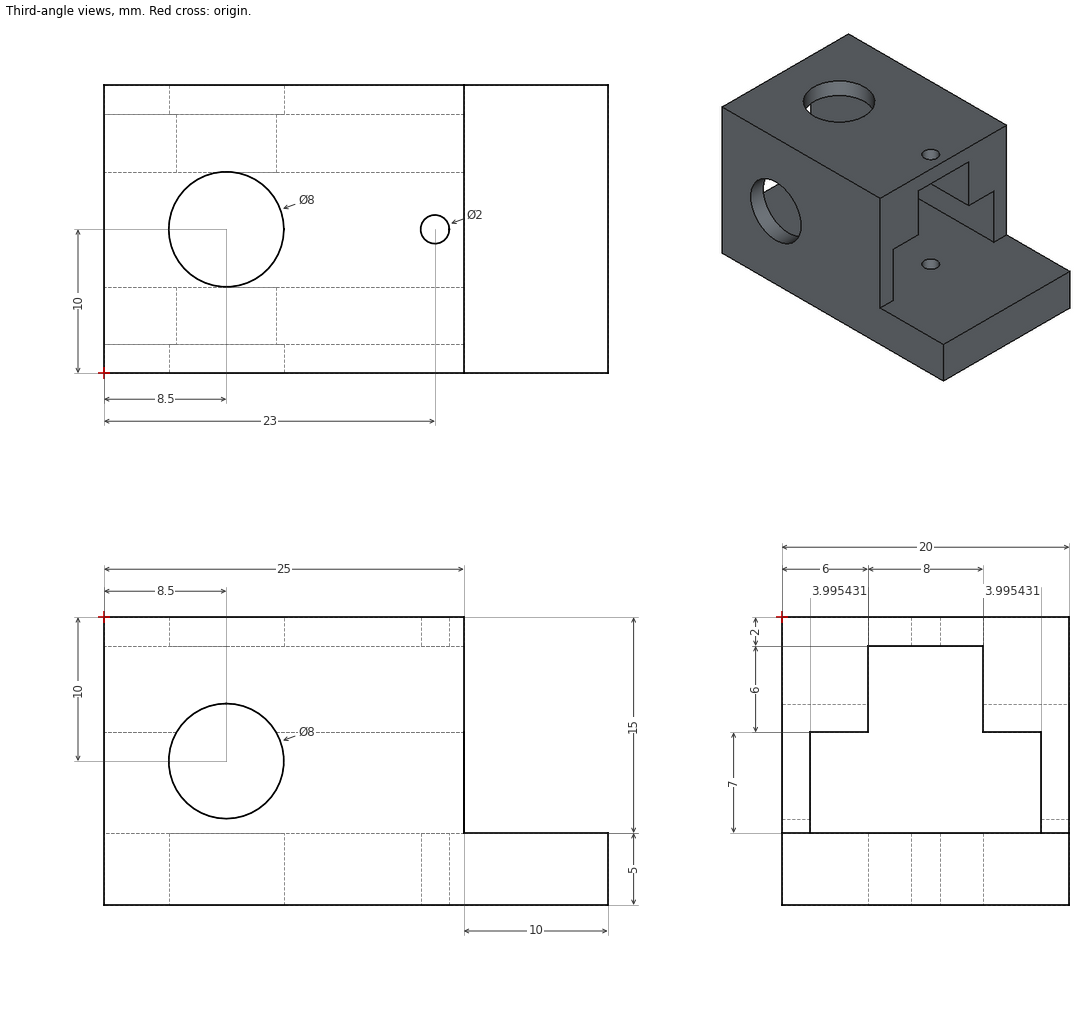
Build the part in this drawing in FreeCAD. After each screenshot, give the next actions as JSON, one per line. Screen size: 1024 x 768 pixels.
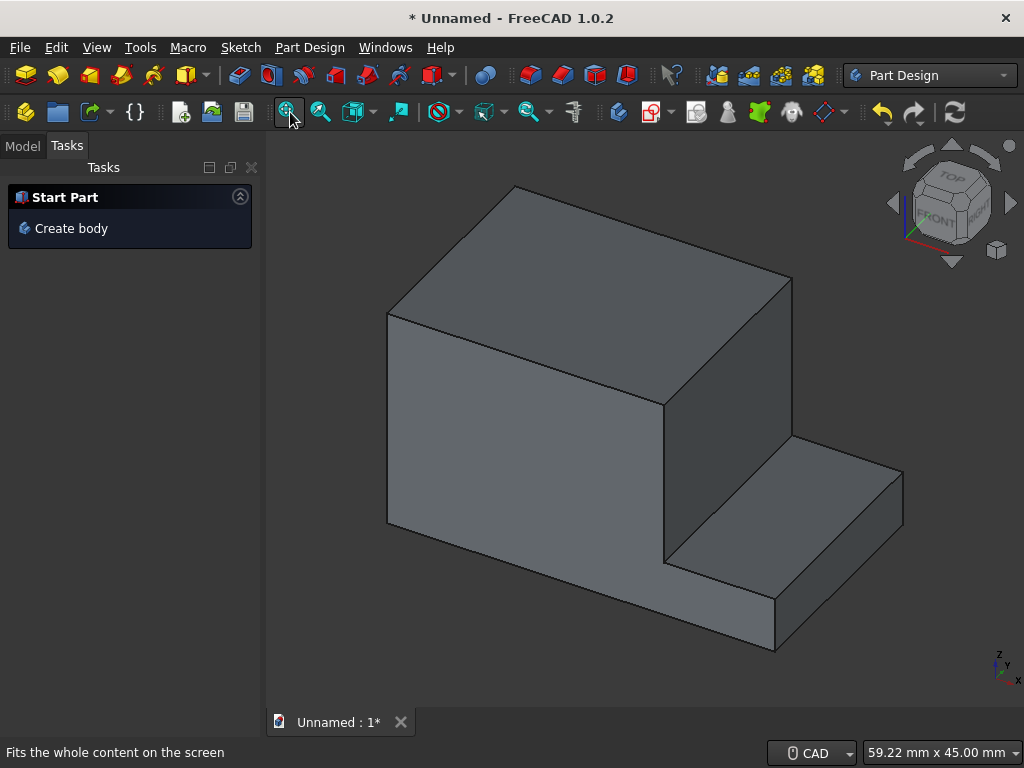
{"action": "left_click", "coordinate": [652, 112]}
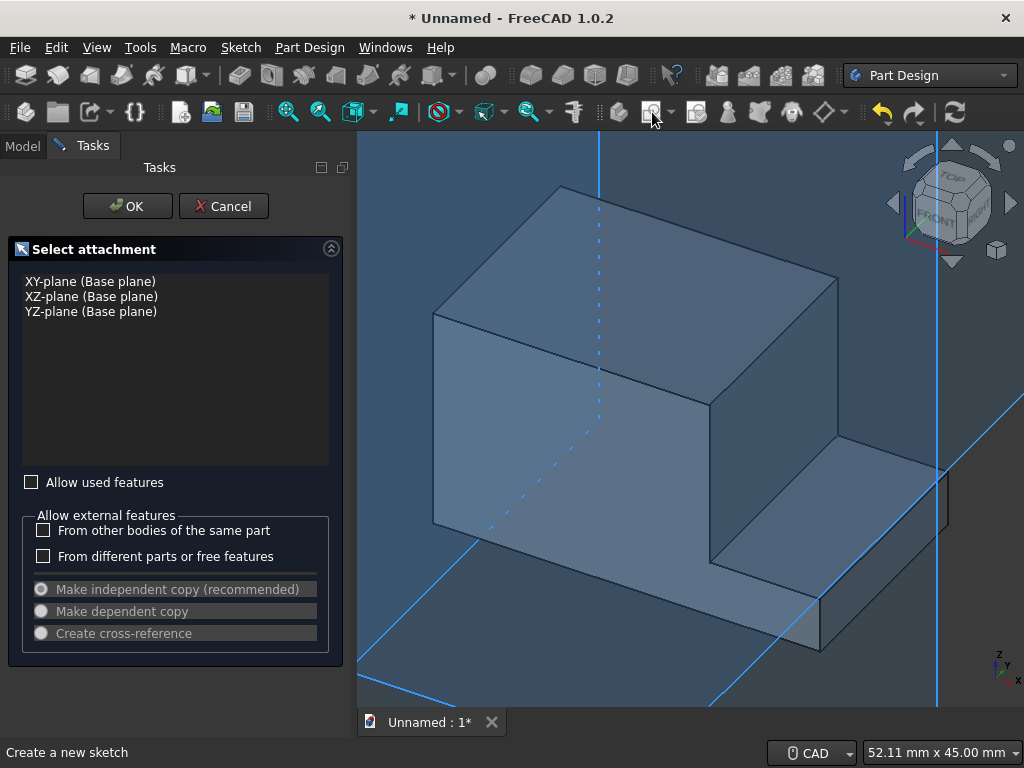
{"action": "left_click", "coordinate": [82, 282]}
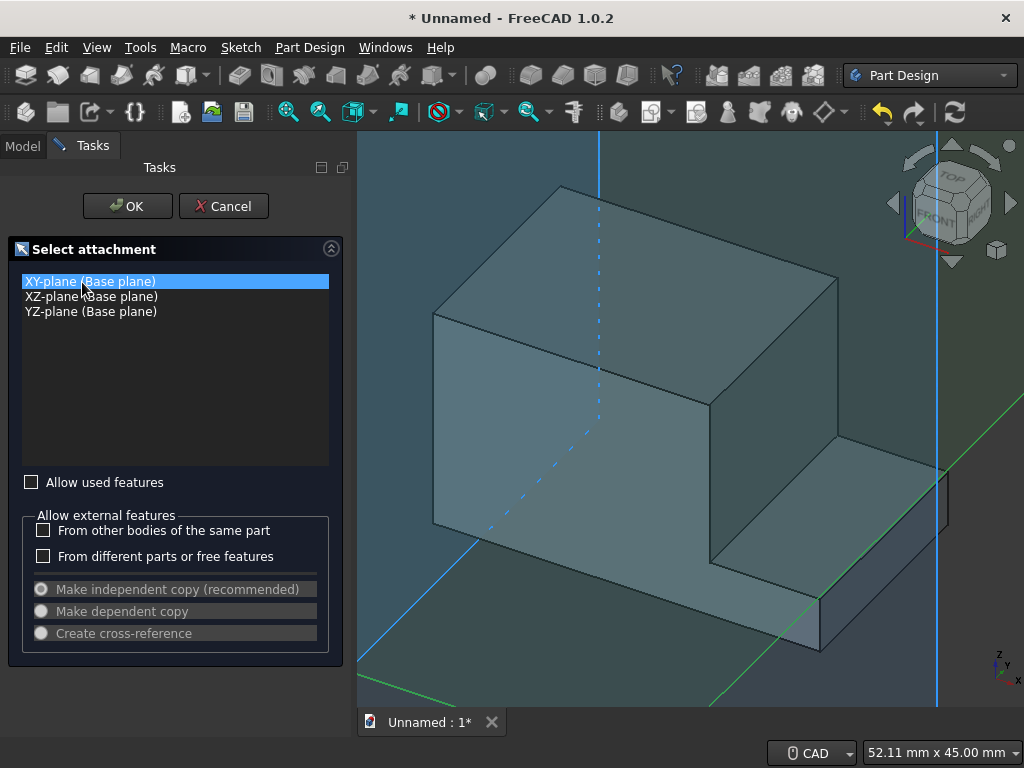
{"action": "left_click", "coordinate": [128, 206]}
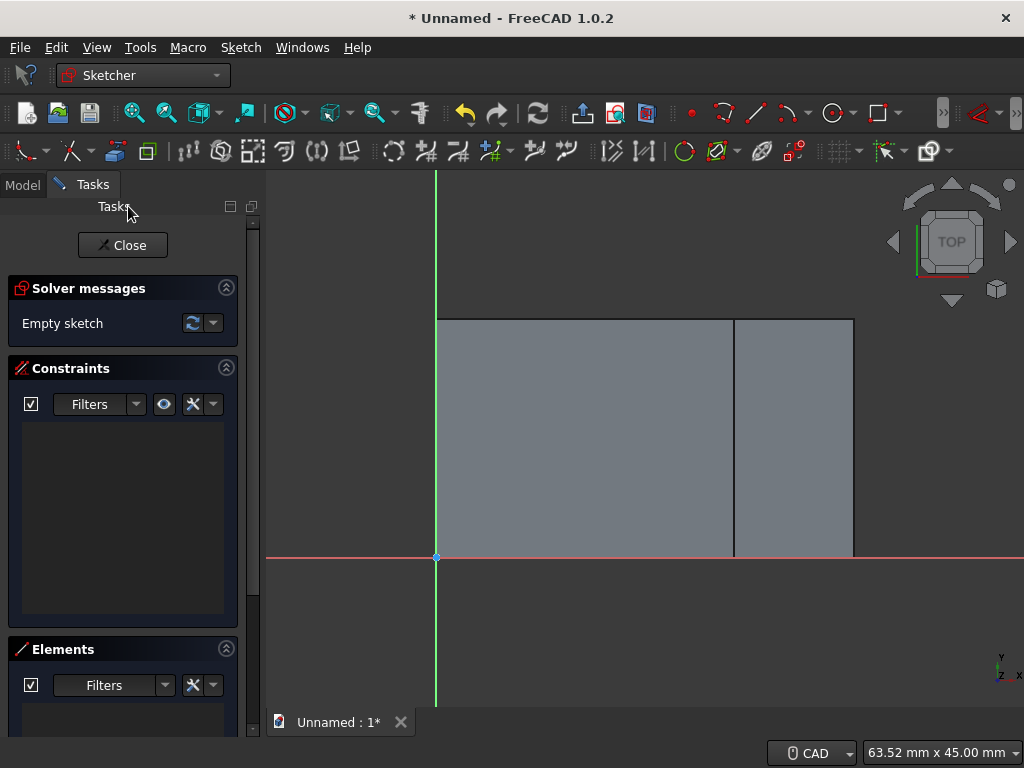
{"action": "scroll", "coordinate": [585, 547], "scroll_direction": "up", "scroll_amount": 2}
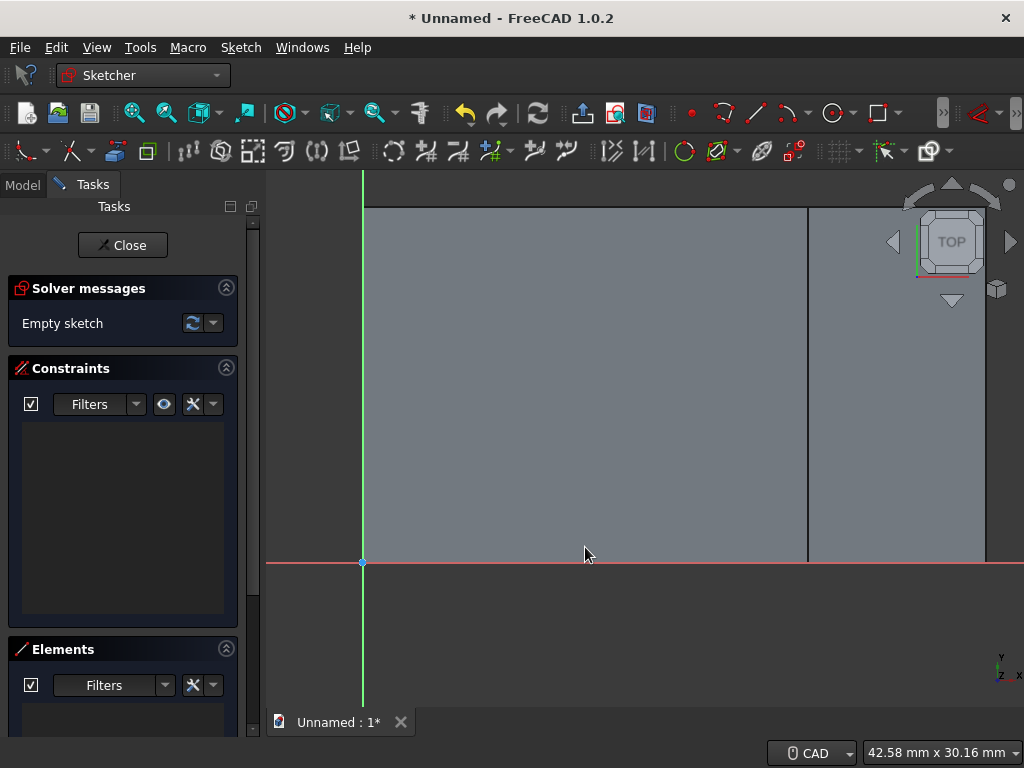
{"action": "key", "text": "g c"}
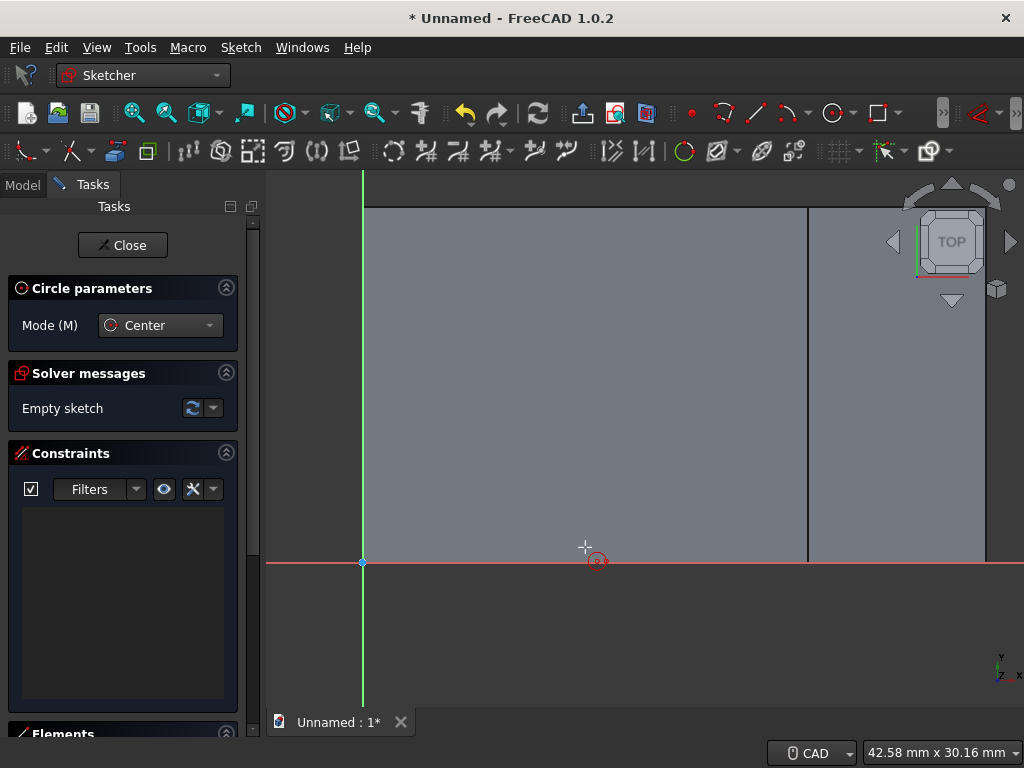
{"action": "left_click", "coordinate": [514, 385]}
{"action": "mouse_move", "coordinate": [564, 334]}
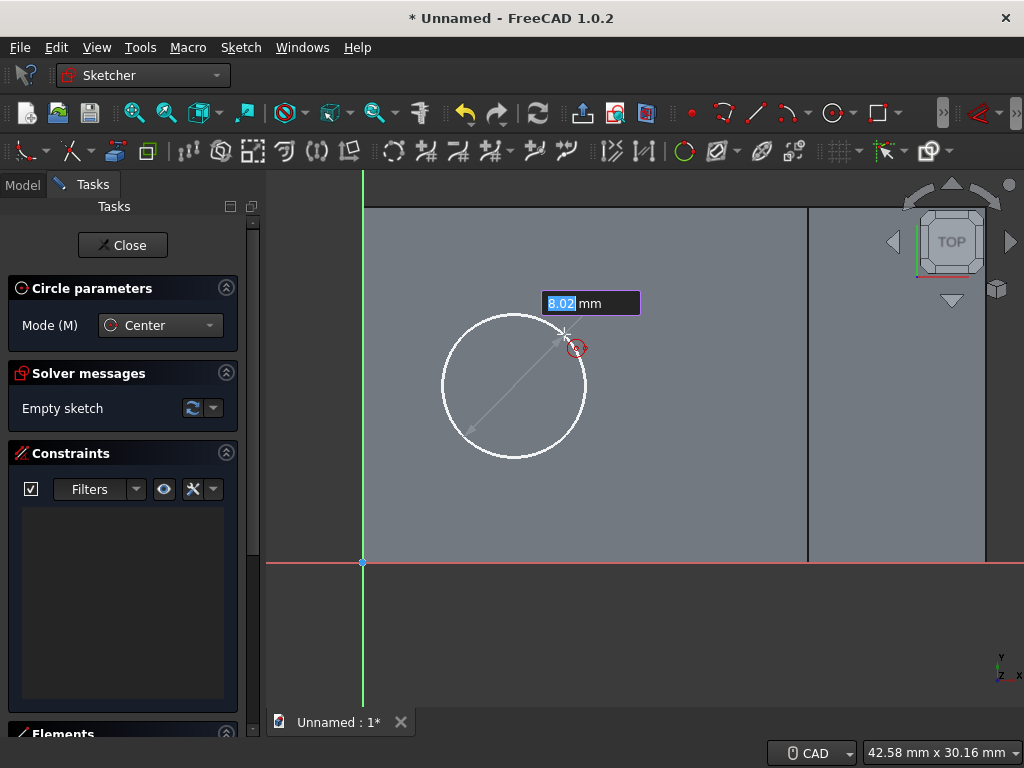
{"action": "type", "text": "8"}
{"action": "key", "text": "Return"}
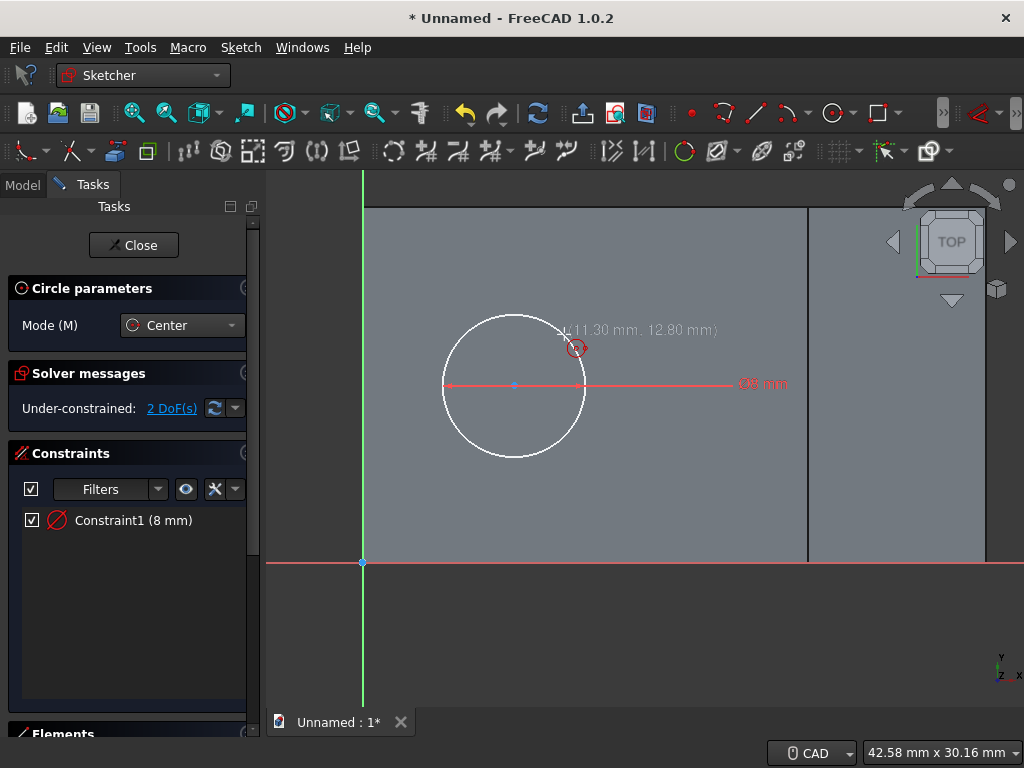
{"action": "scroll", "coordinate": [772, 385], "scroll_direction": "up", "scroll_amount": 2}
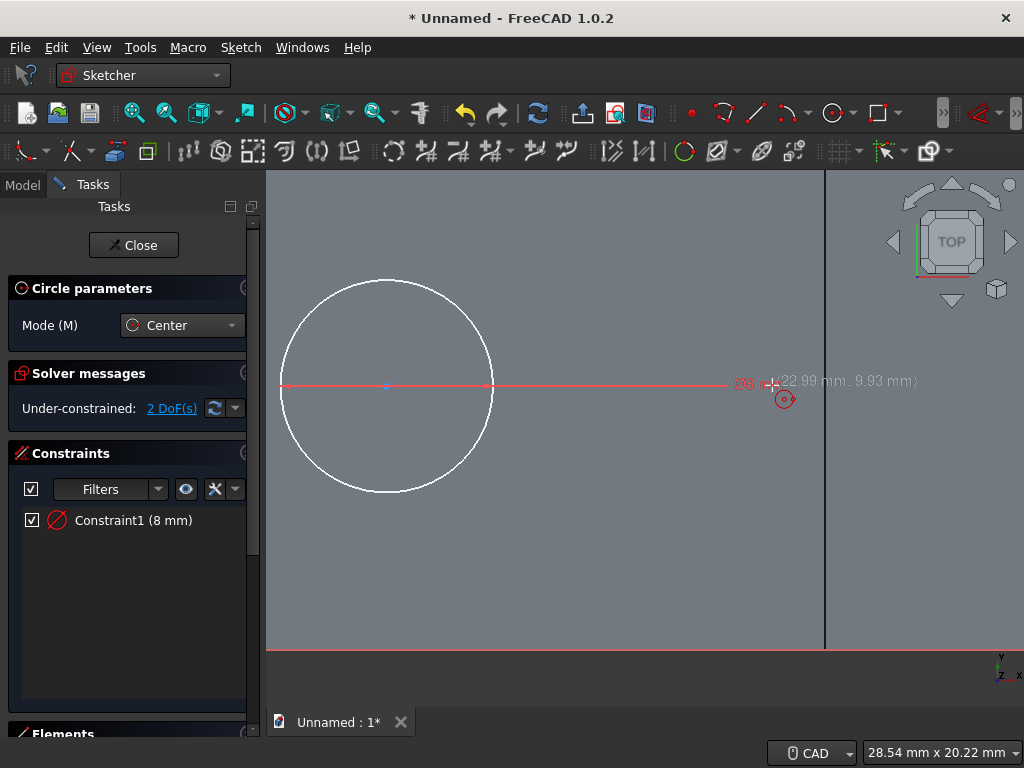
{"action": "left_click", "coordinate": [772, 384]}
{"action": "mouse_move", "coordinate": [791, 366]}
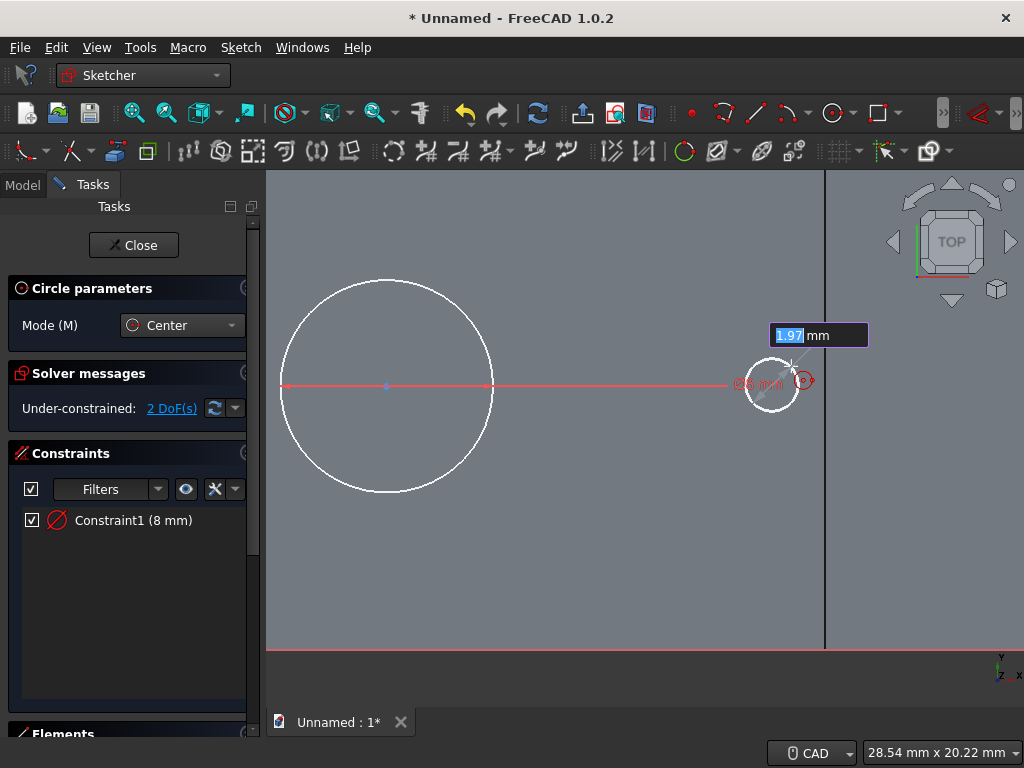
{"action": "type", "text": "2"}
{"action": "key", "text": "Return"}
{"action": "key", "text": "Escape"}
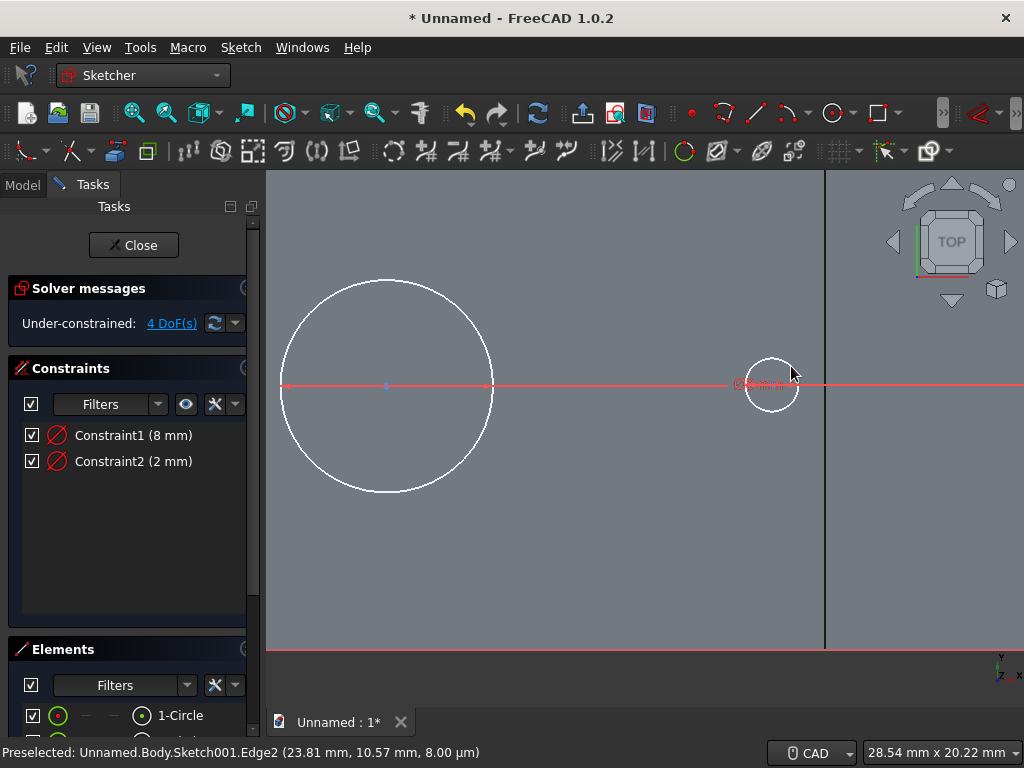
{"action": "left_click", "coordinate": [387, 386]}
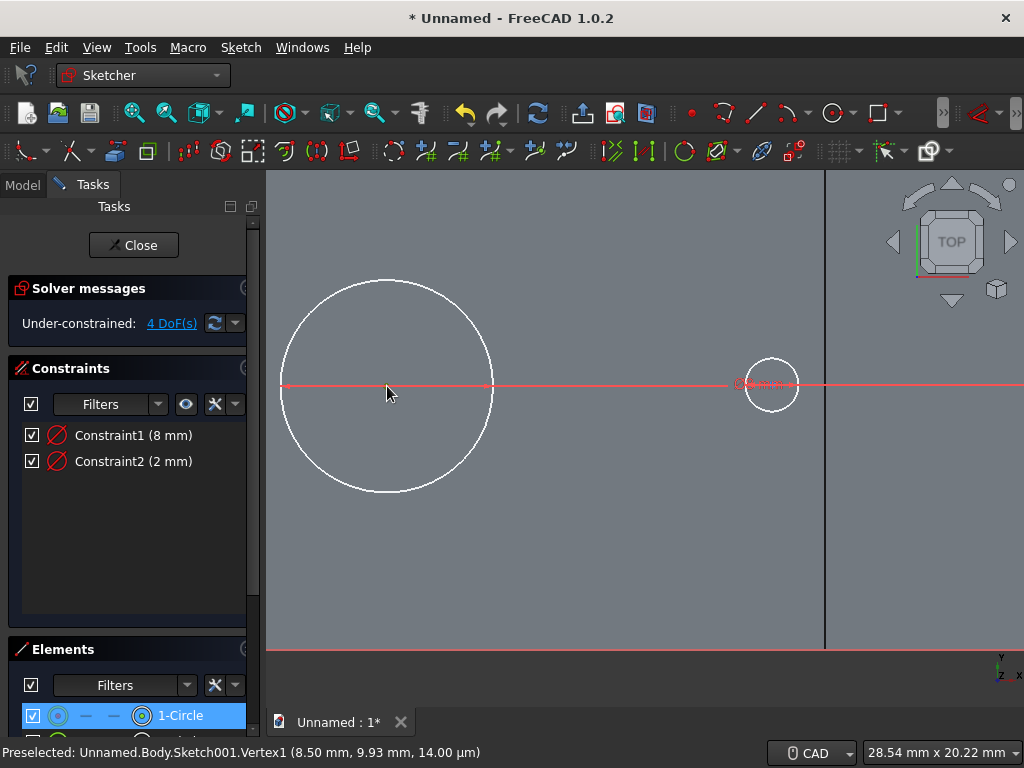
{"action": "left_click", "coordinate": [772, 385]}